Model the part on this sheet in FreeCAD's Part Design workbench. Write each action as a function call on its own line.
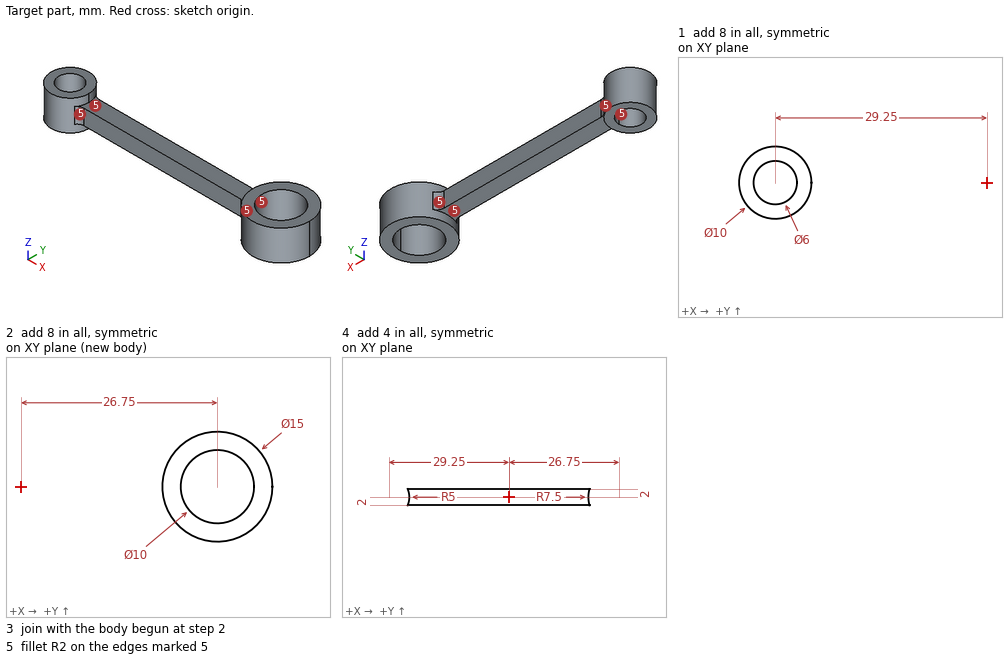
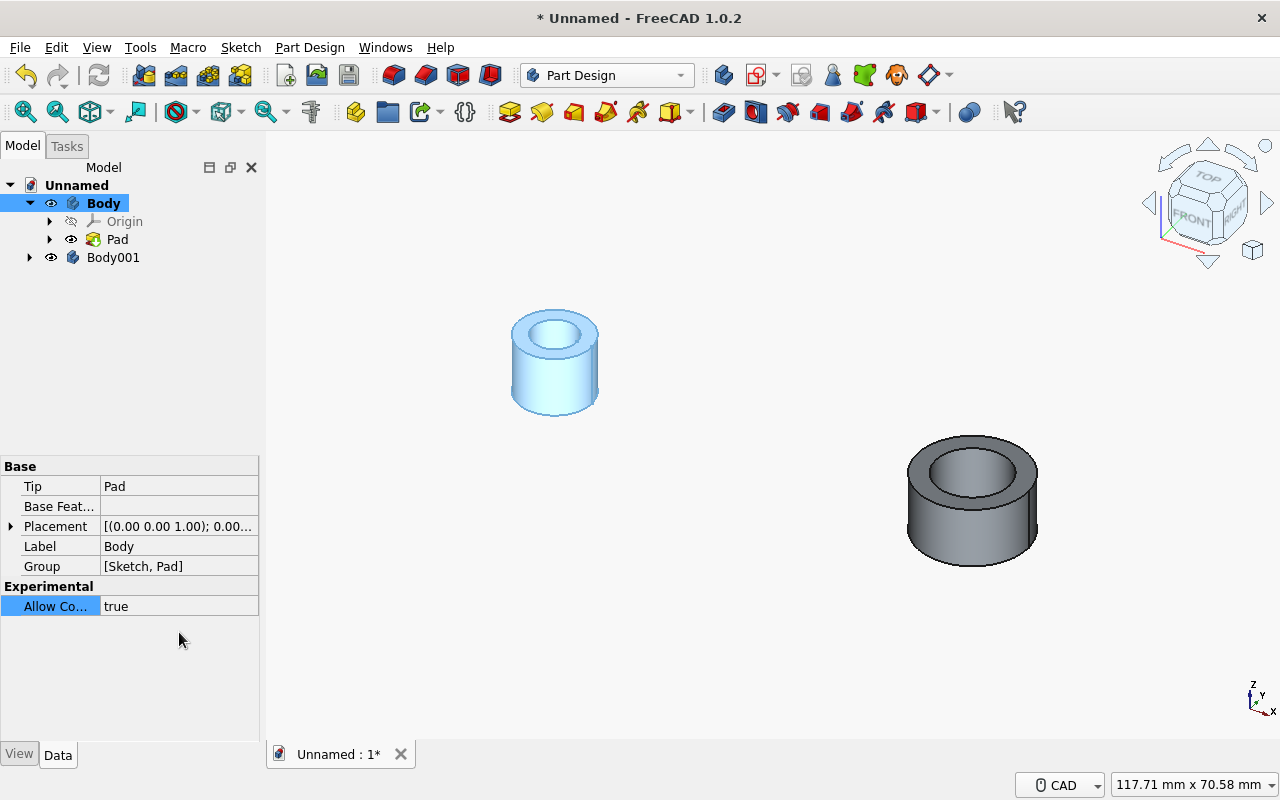
click(96, 257)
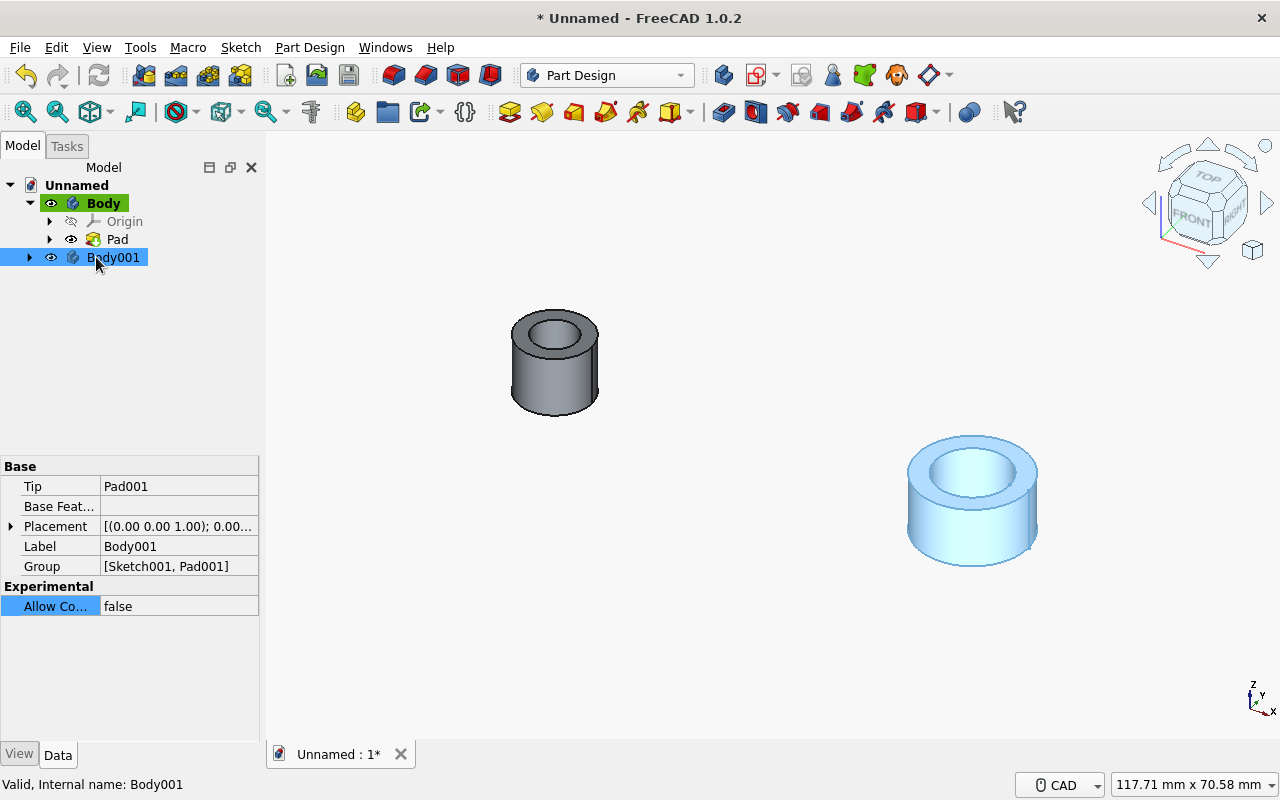
click(970, 112)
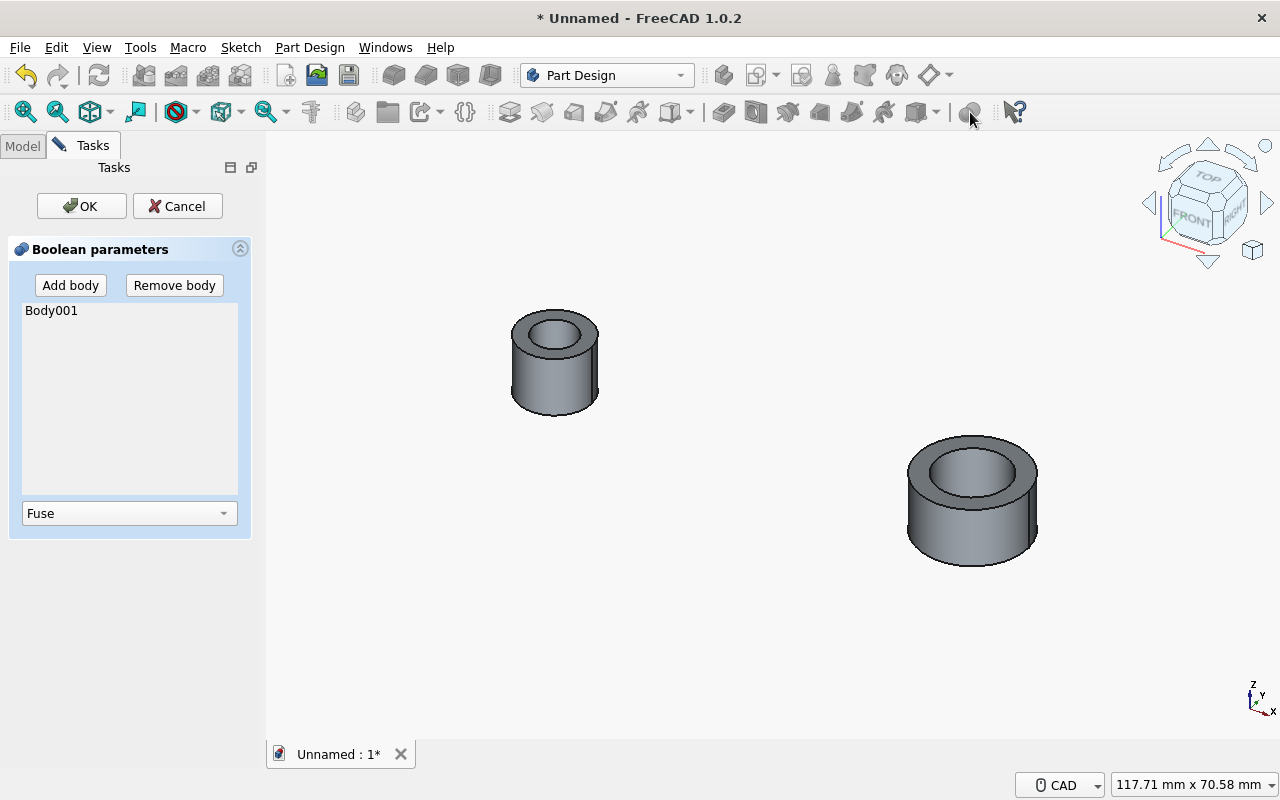
click(82, 206)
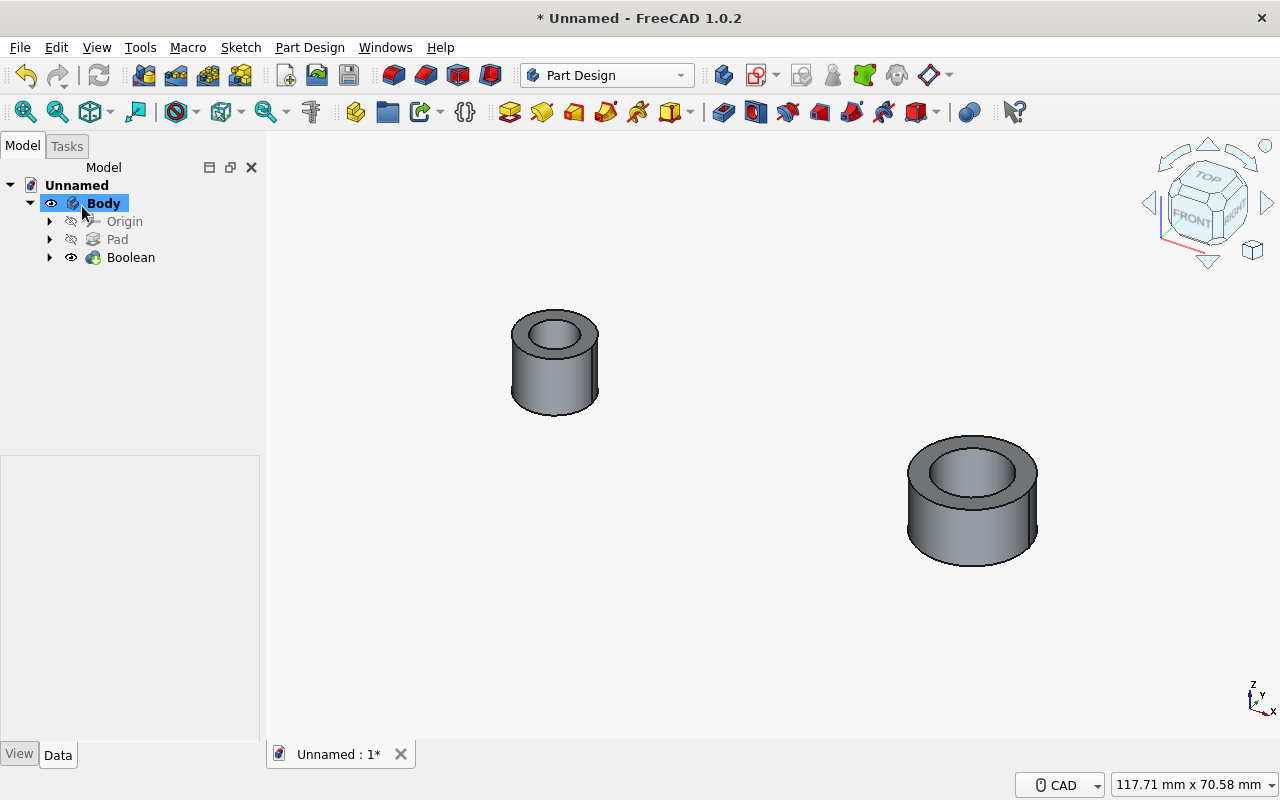
click(756, 76)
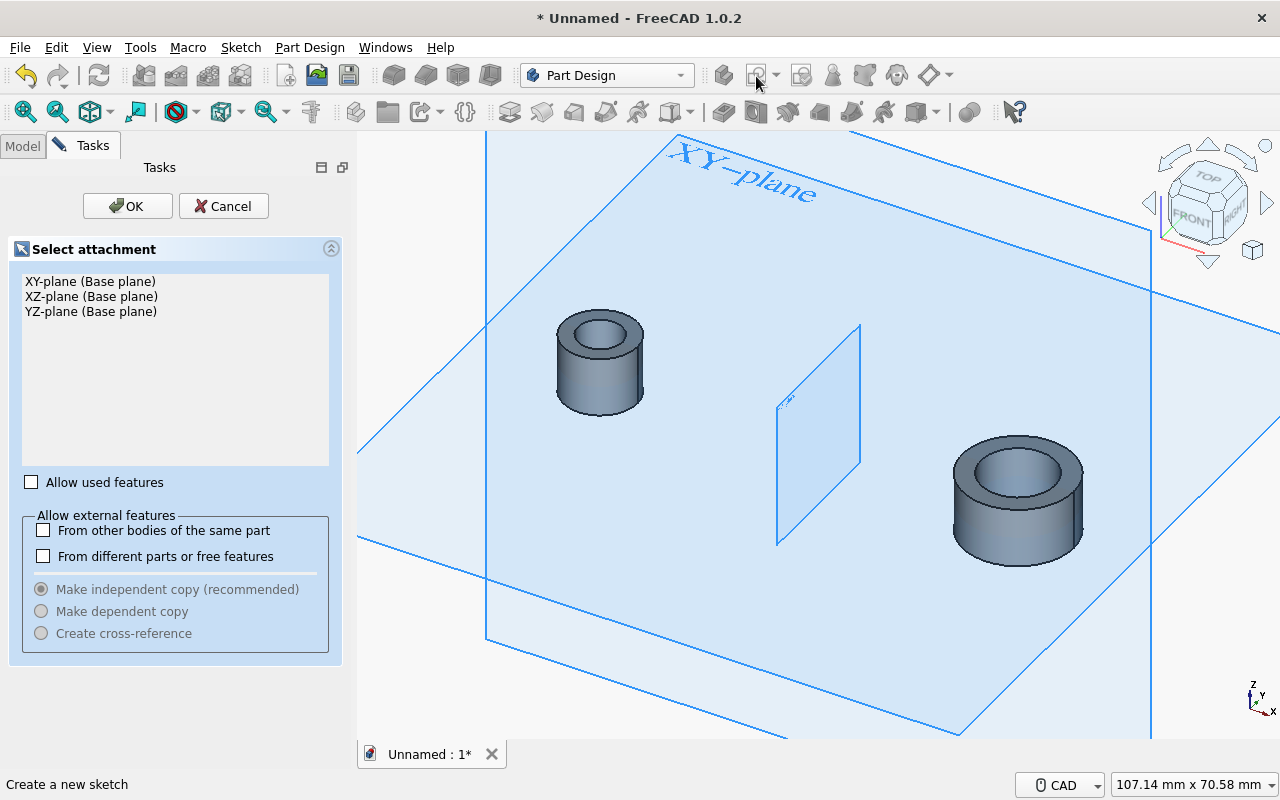
click(82, 282)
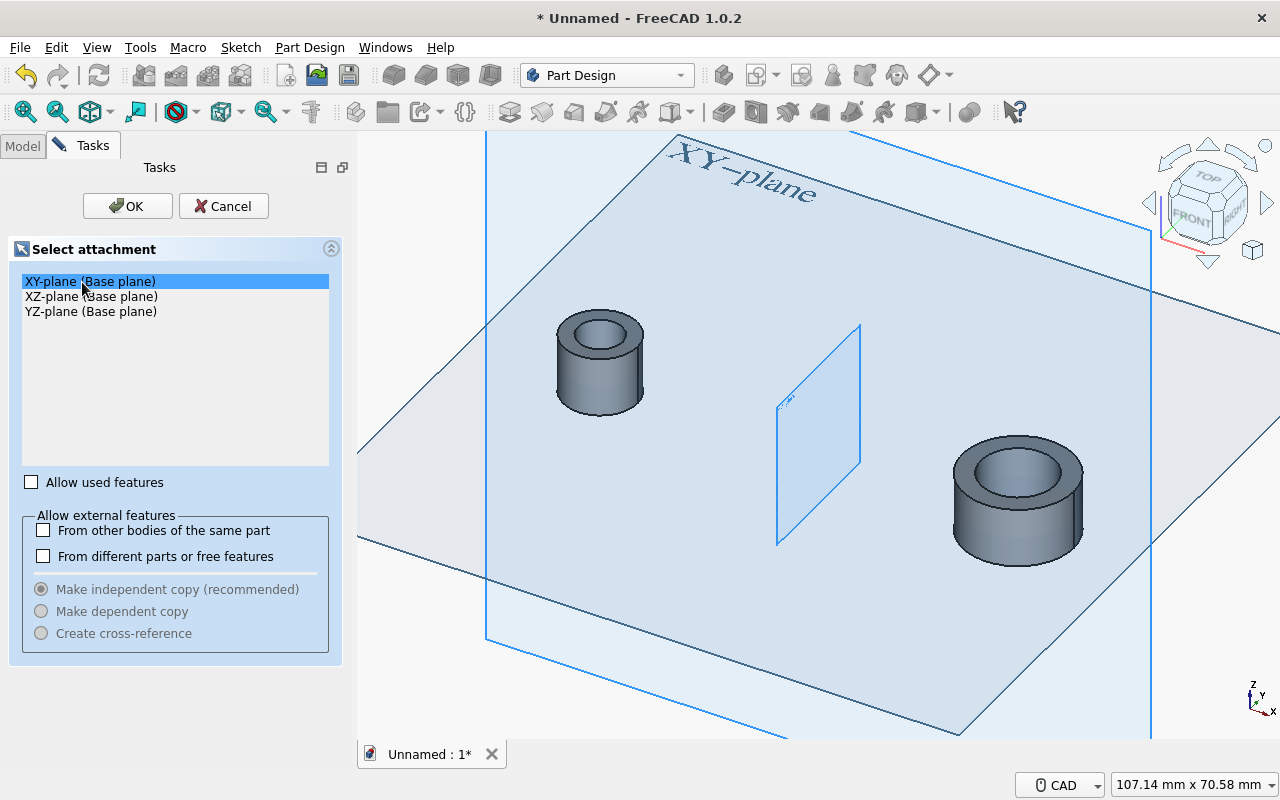
click(128, 206)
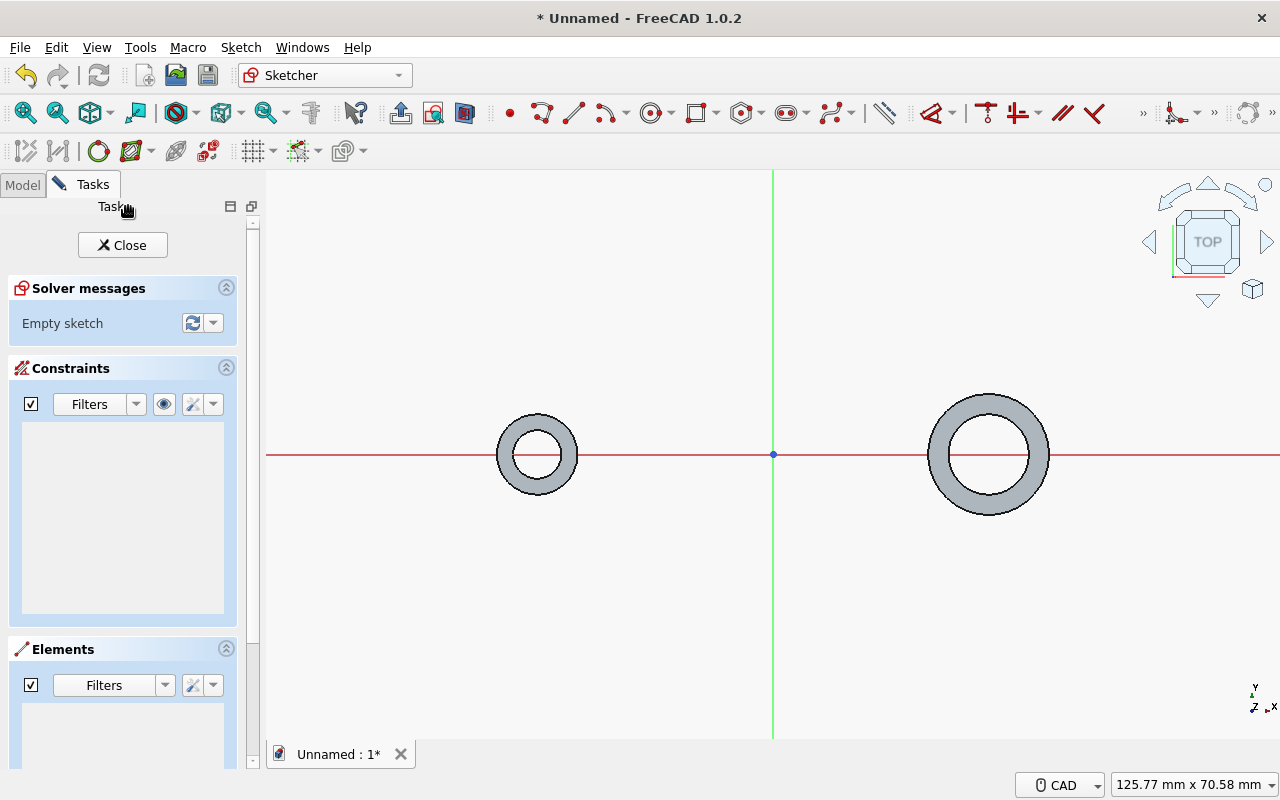
click(466, 114)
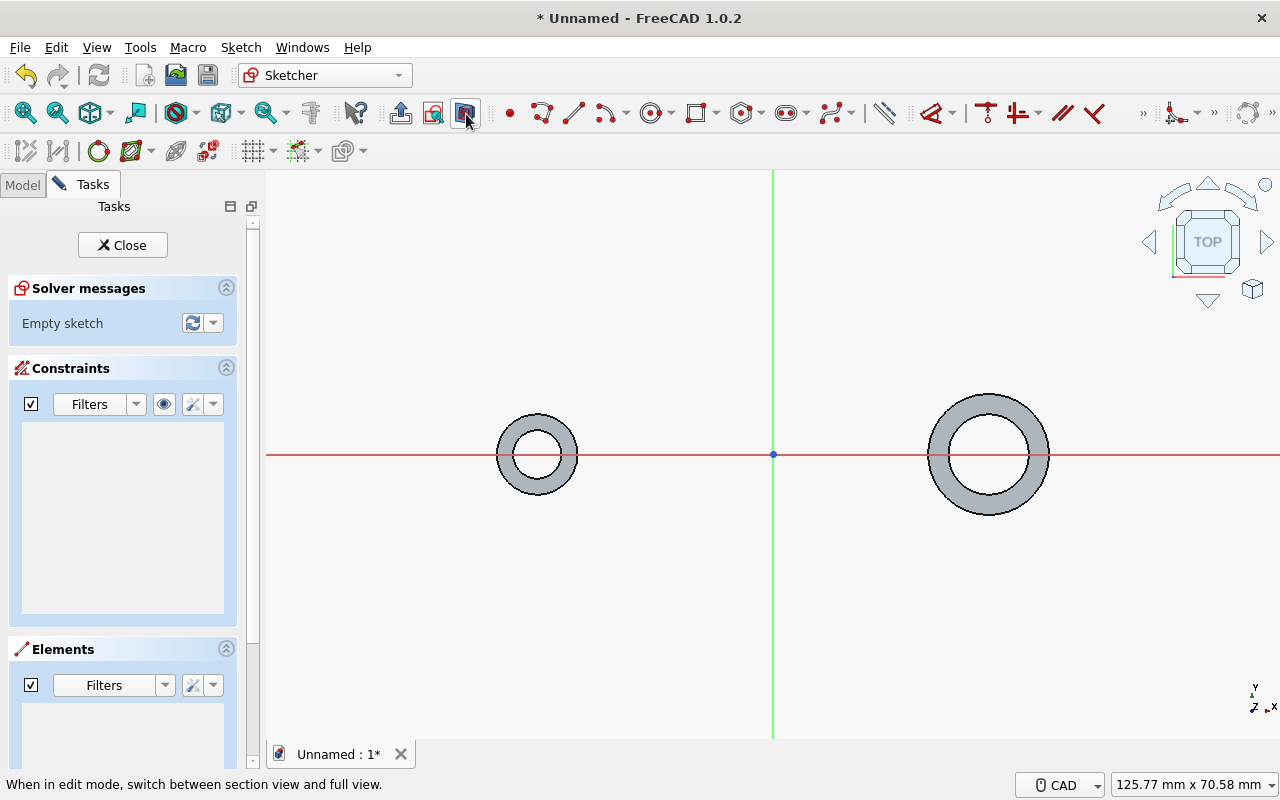
scroll(849, 455, up, 2)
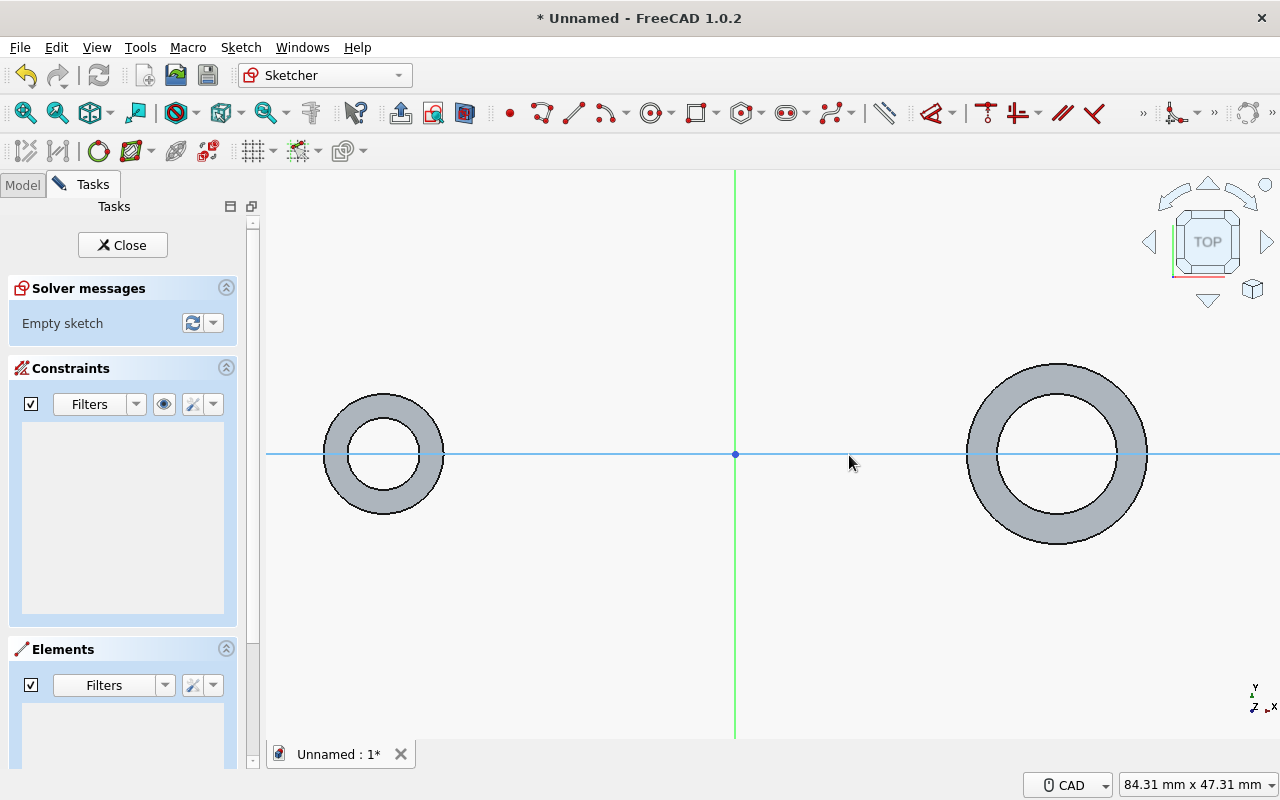
click(574, 114)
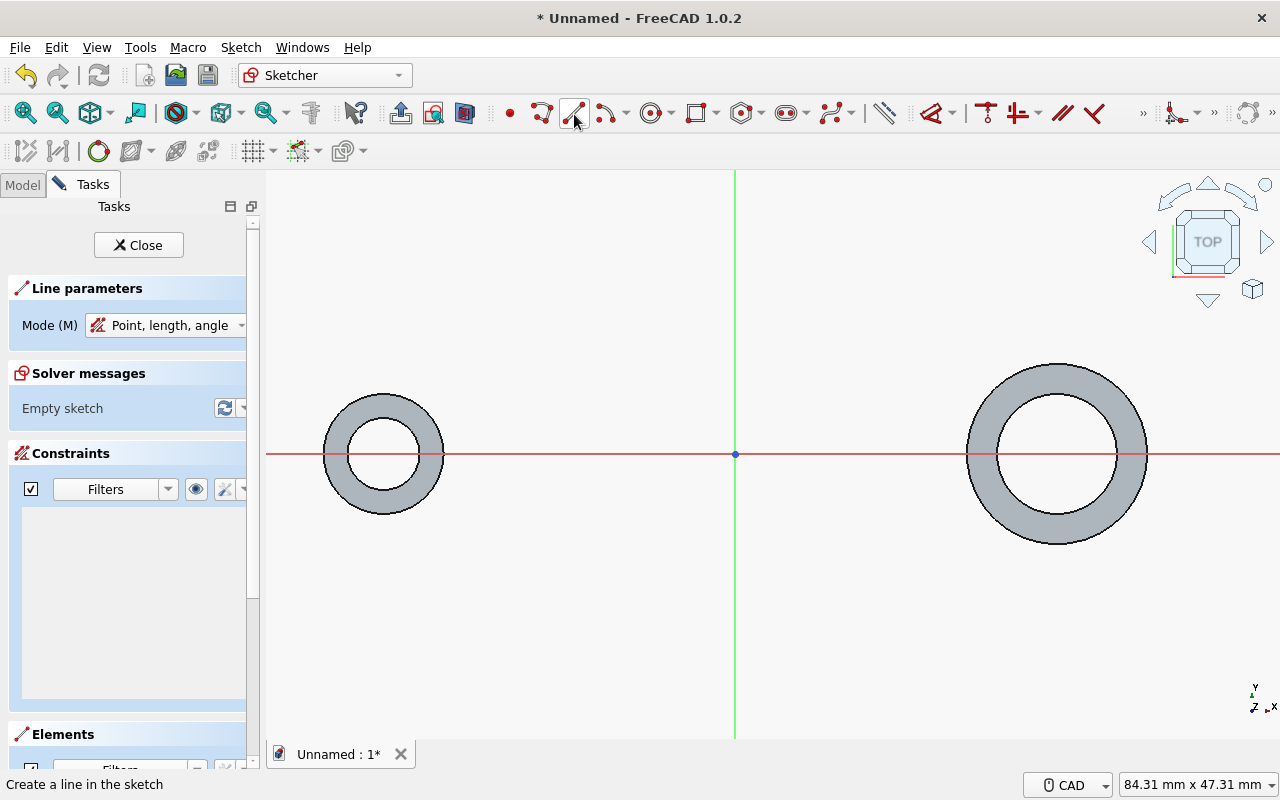
click(970, 430)
click(439, 430)